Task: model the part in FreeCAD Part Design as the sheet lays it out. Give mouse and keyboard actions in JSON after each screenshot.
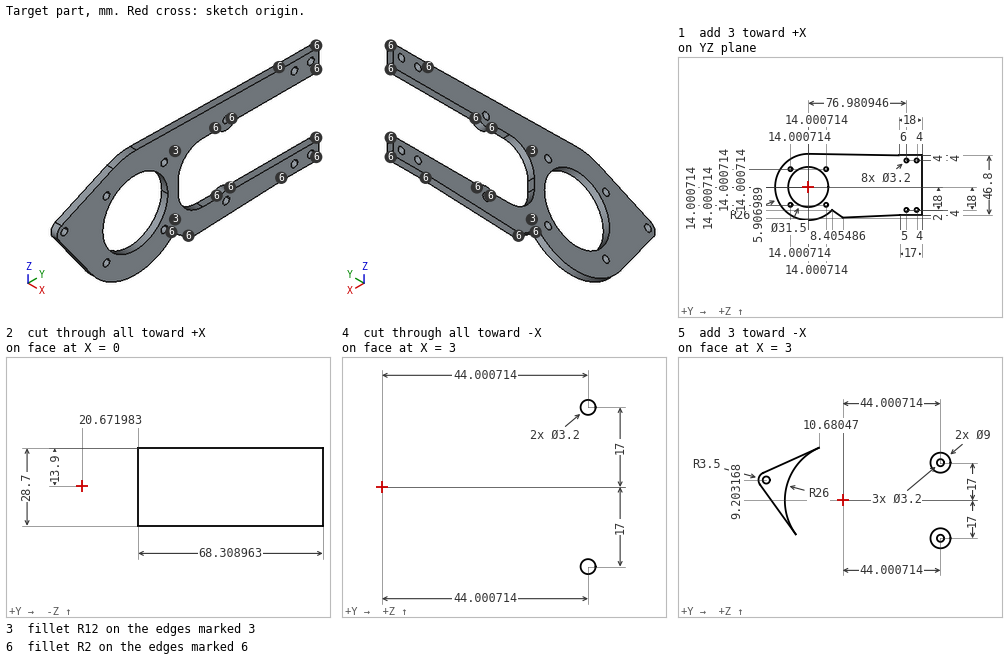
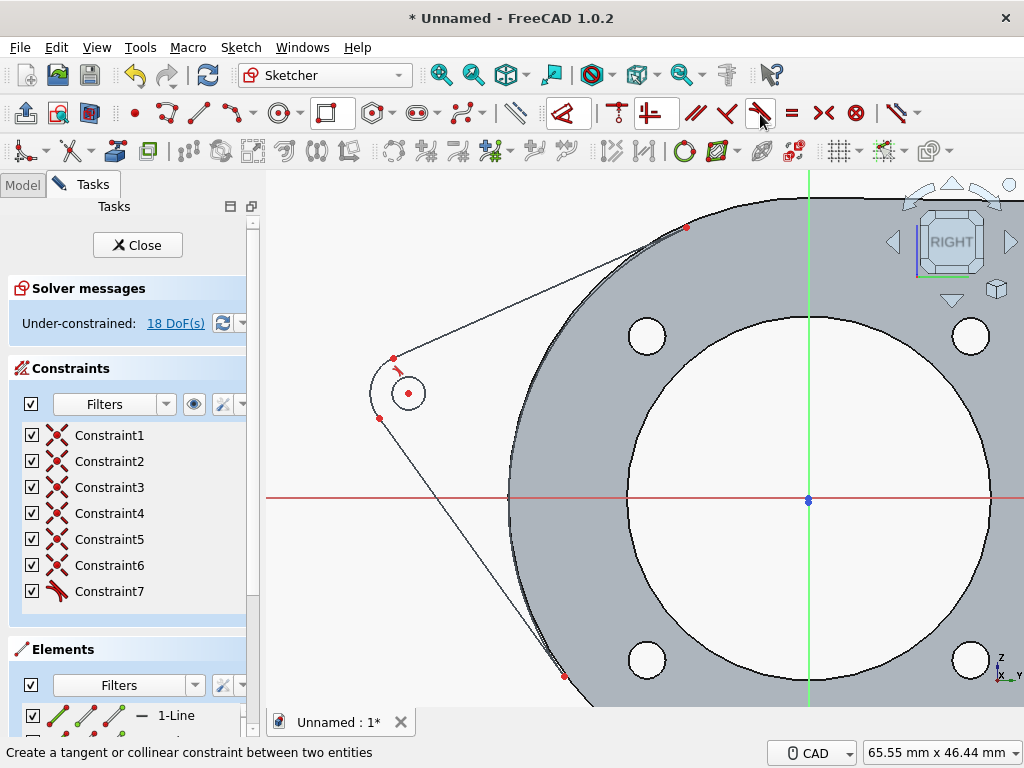
{"action": "left_click", "coordinate": [599, 267]}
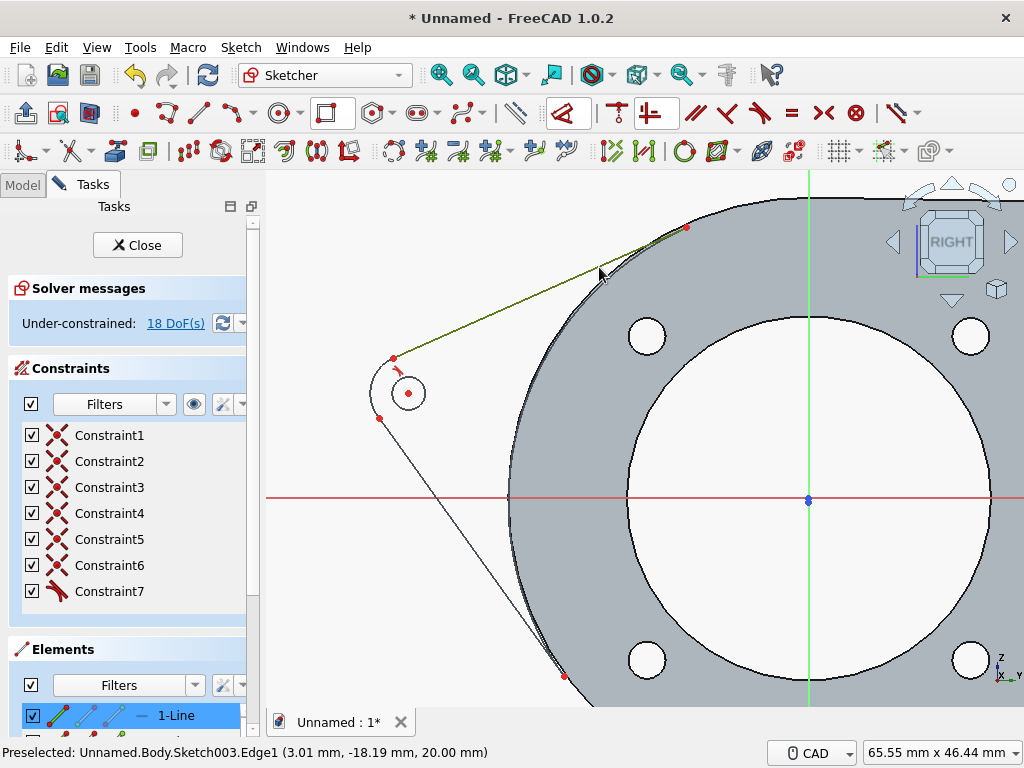
{"action": "left_click", "coordinate": [564, 328]}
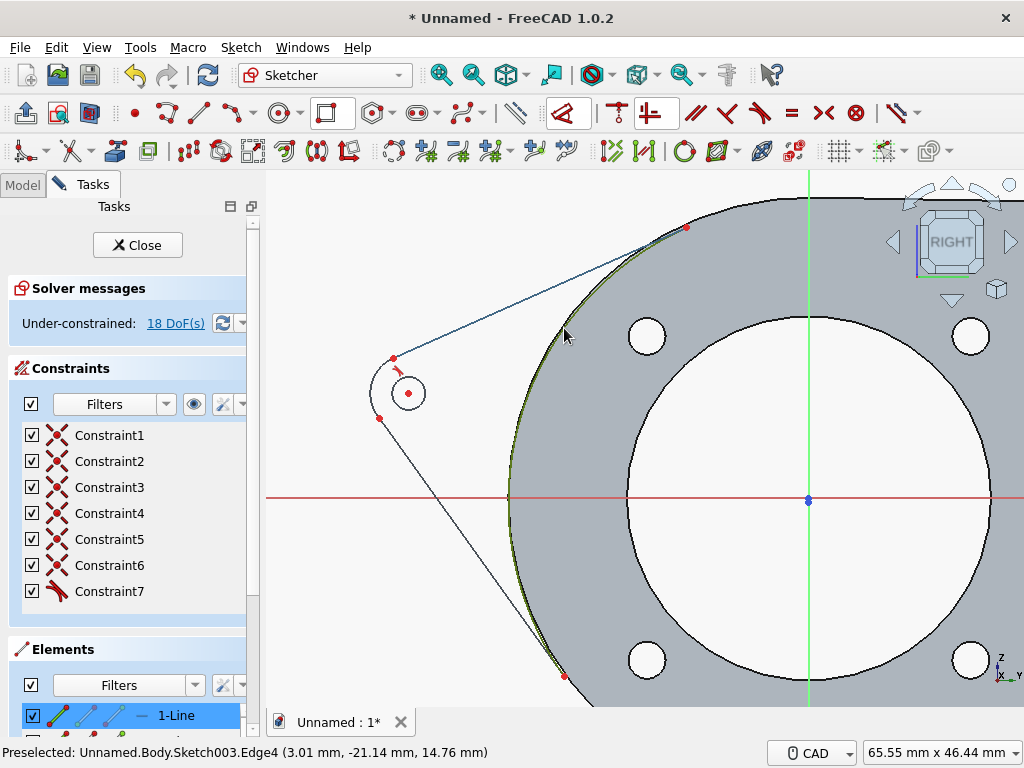
{"action": "left_click", "coordinate": [760, 114]}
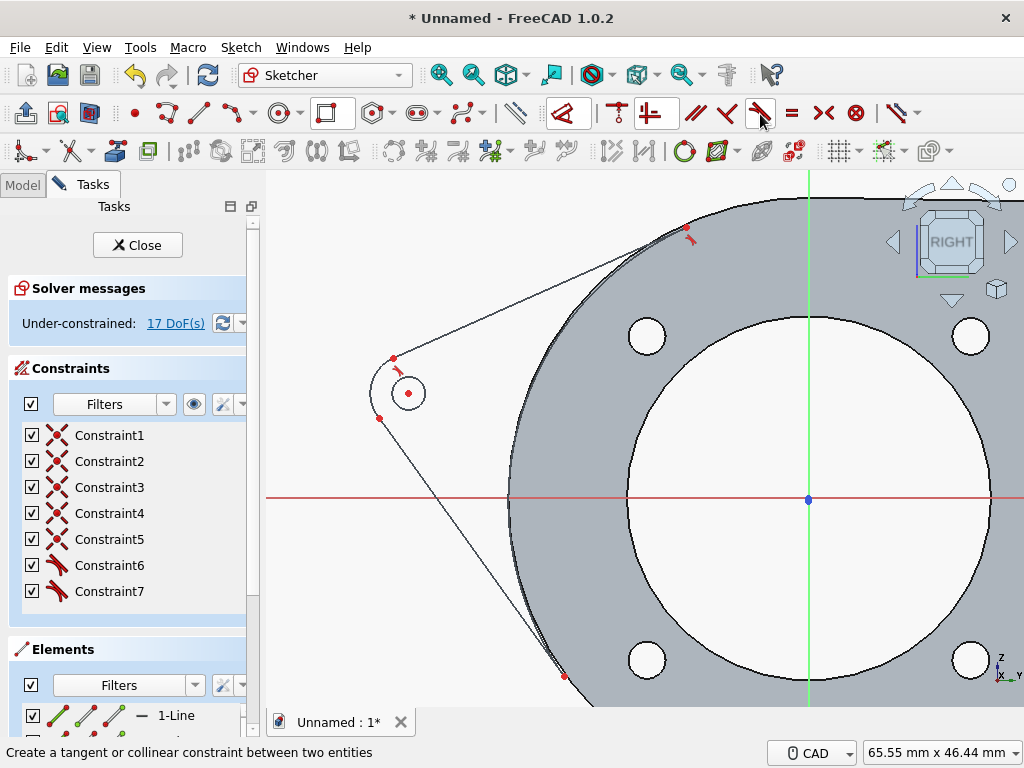
{"action": "left_click", "coordinate": [435, 496]}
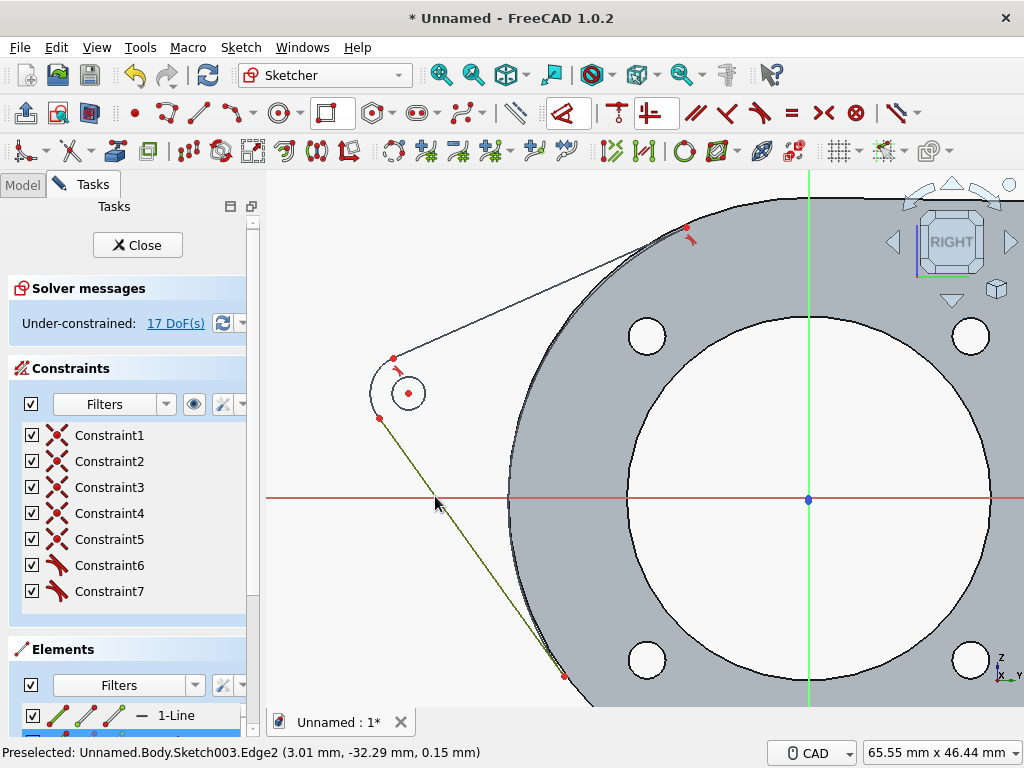
{"action": "left_click", "coordinate": [377, 372]}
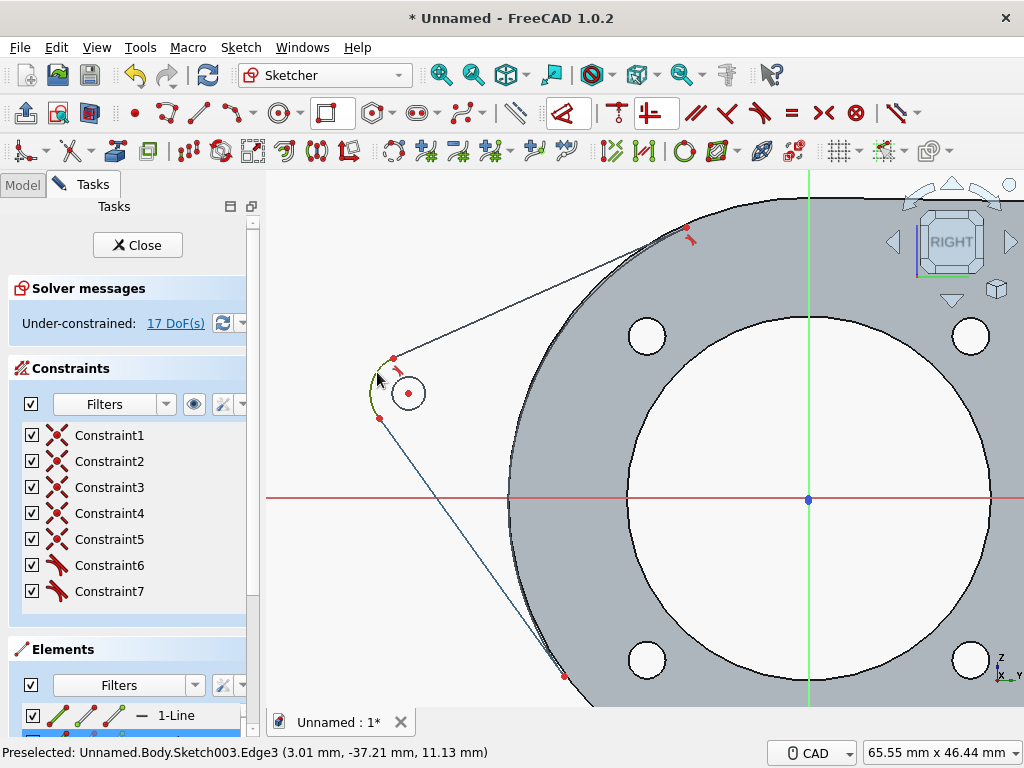
{"action": "left_click", "coordinate": [760, 114]}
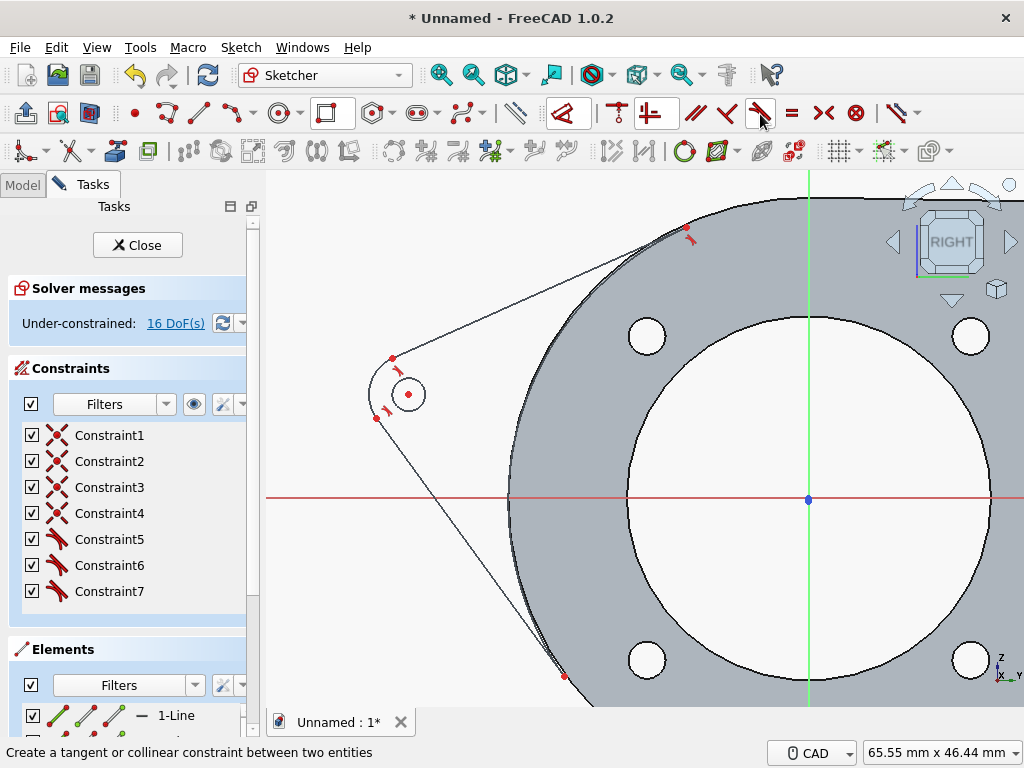
{"action": "left_click", "coordinate": [433, 496]}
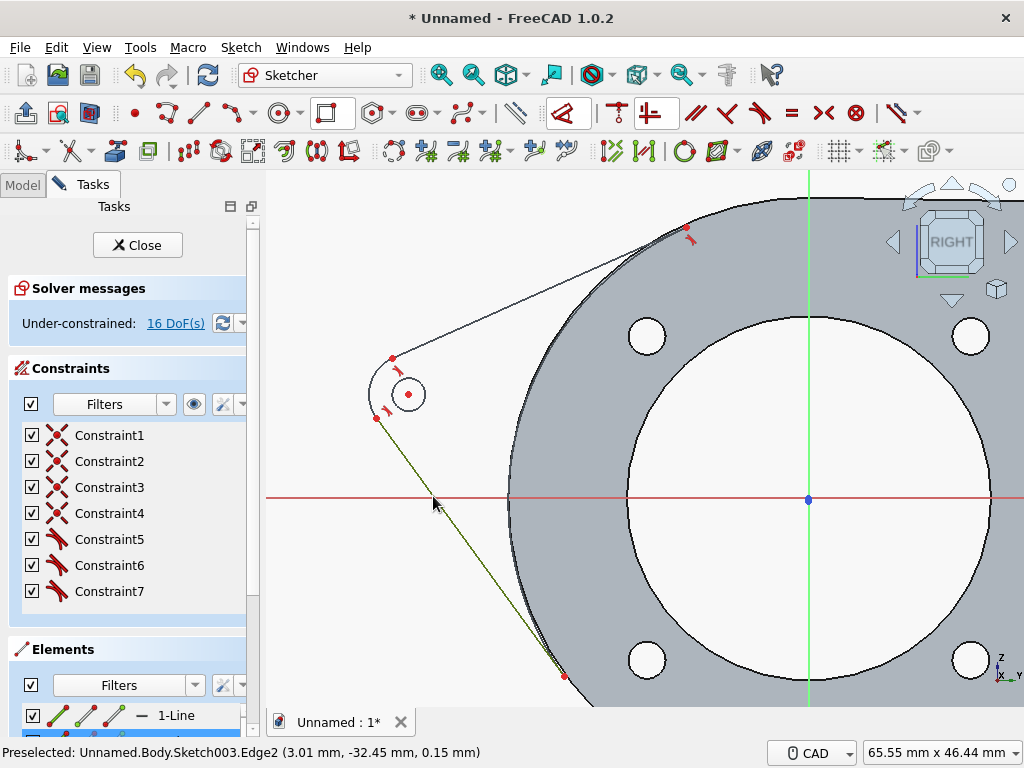
{"action": "left_click", "coordinate": [564, 327]}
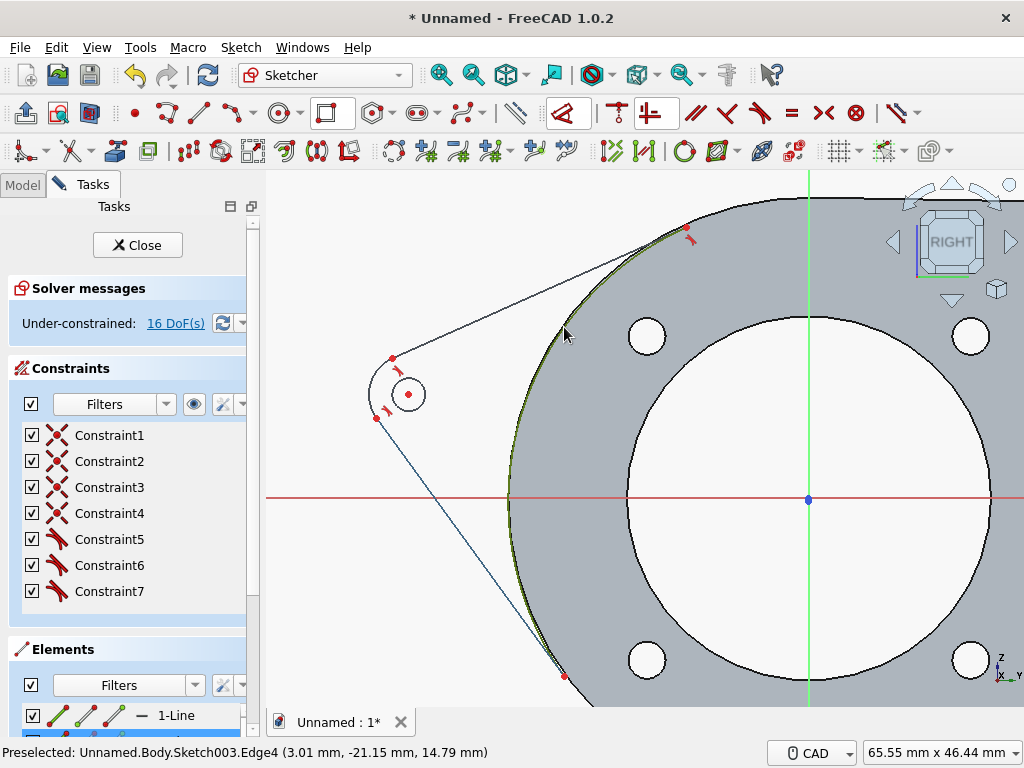
{"action": "left_click", "coordinate": [760, 114]}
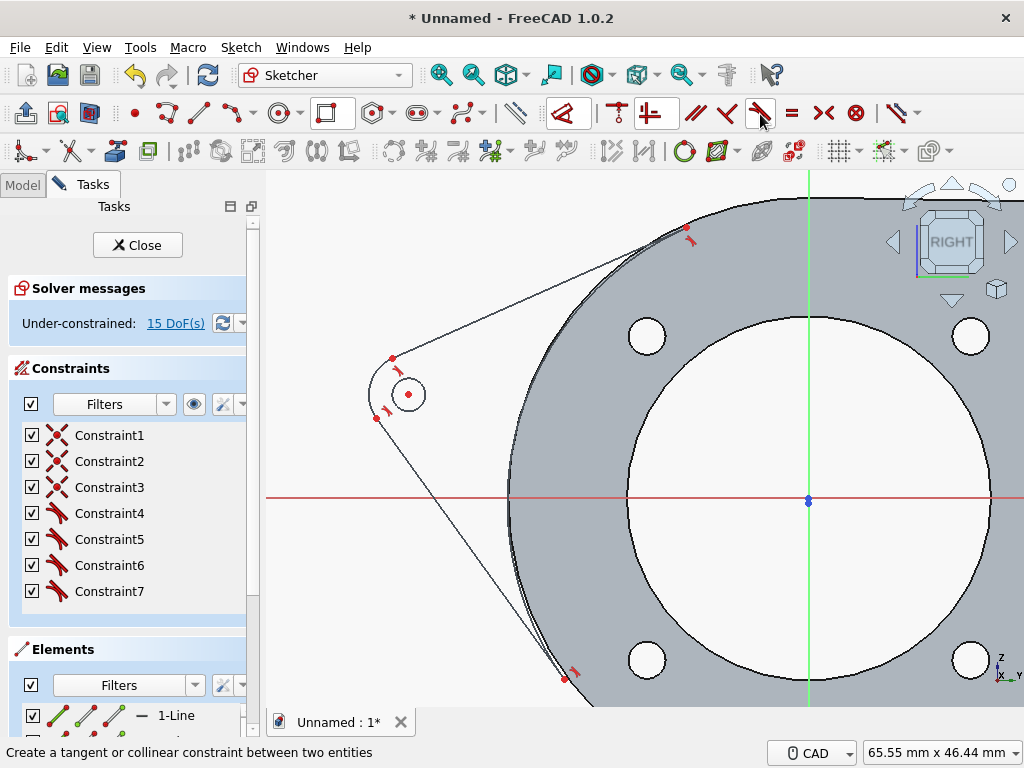
{"action": "scroll", "coordinate": [809, 501], "scroll_direction": "up", "scroll_amount": 5}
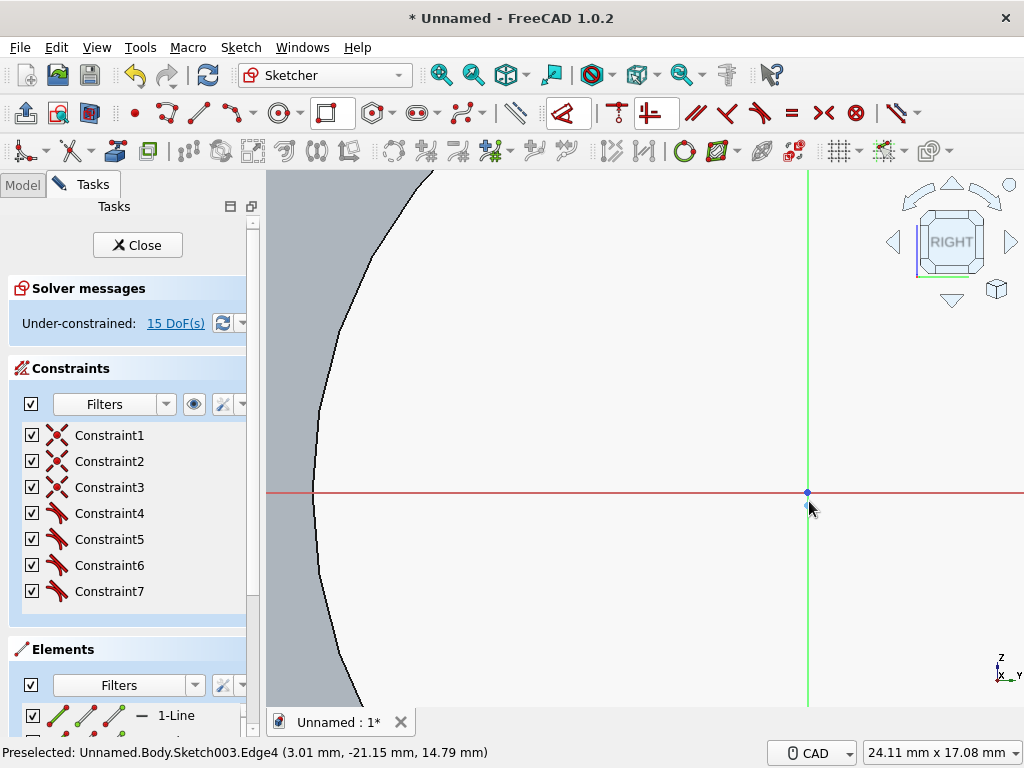
{"action": "left_click_drag", "start_coordinate": [797, 483], "coordinate": [818, 516]}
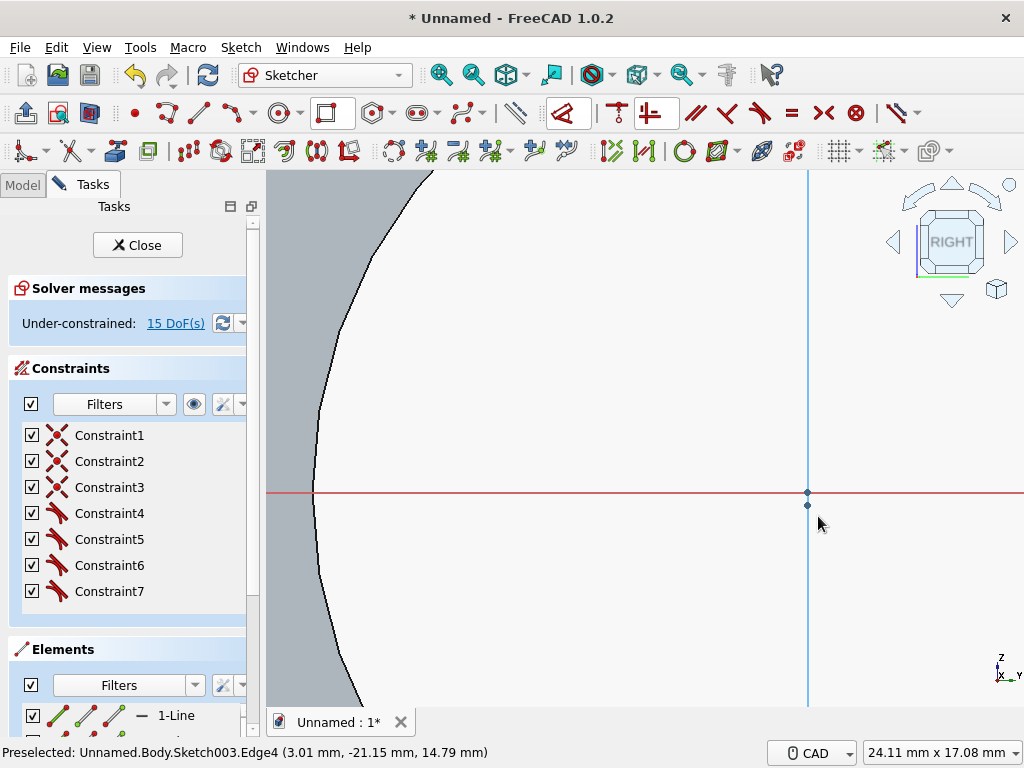
{"action": "left_click", "coordinate": [618, 114]}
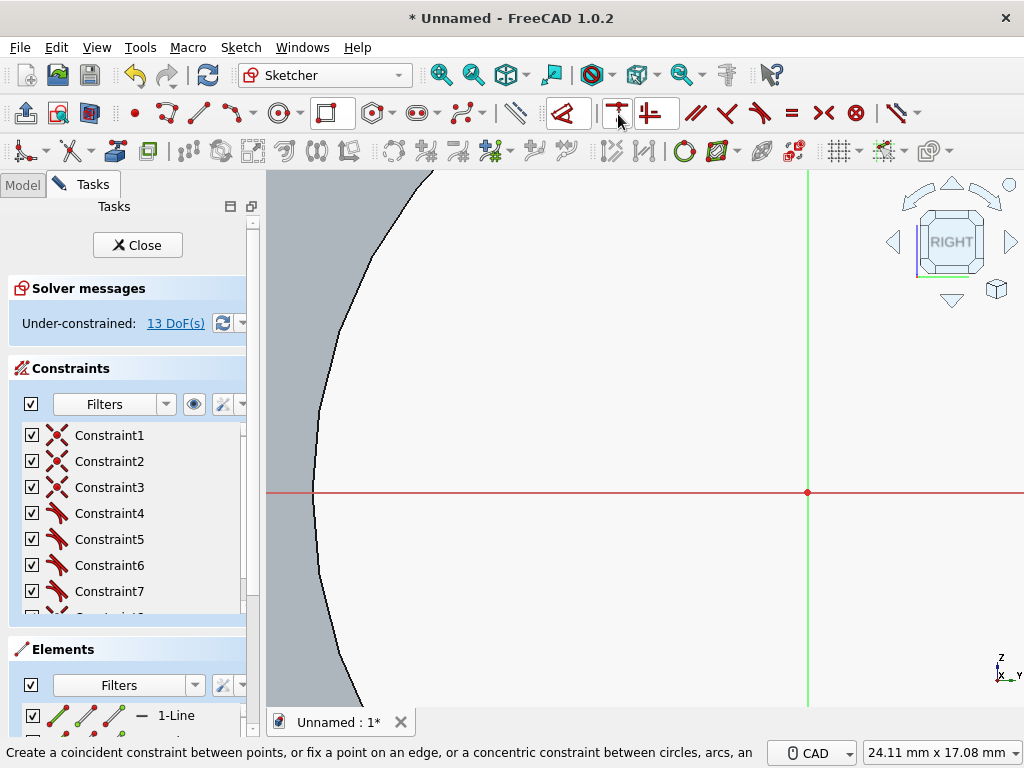
{"action": "scroll", "coordinate": [514, 435], "scroll_direction": "down", "scroll_amount": 10}